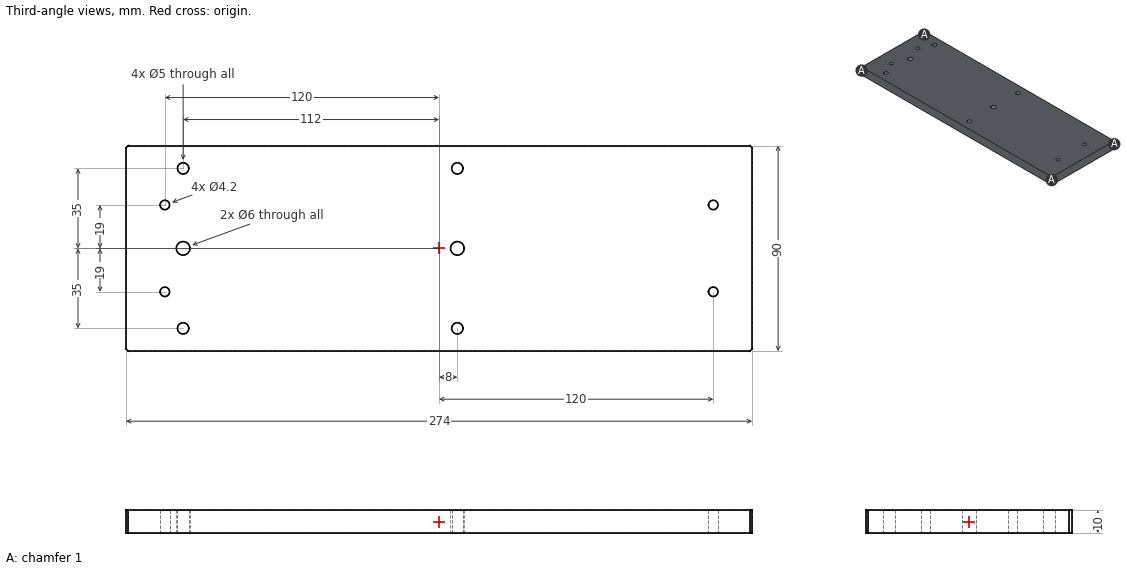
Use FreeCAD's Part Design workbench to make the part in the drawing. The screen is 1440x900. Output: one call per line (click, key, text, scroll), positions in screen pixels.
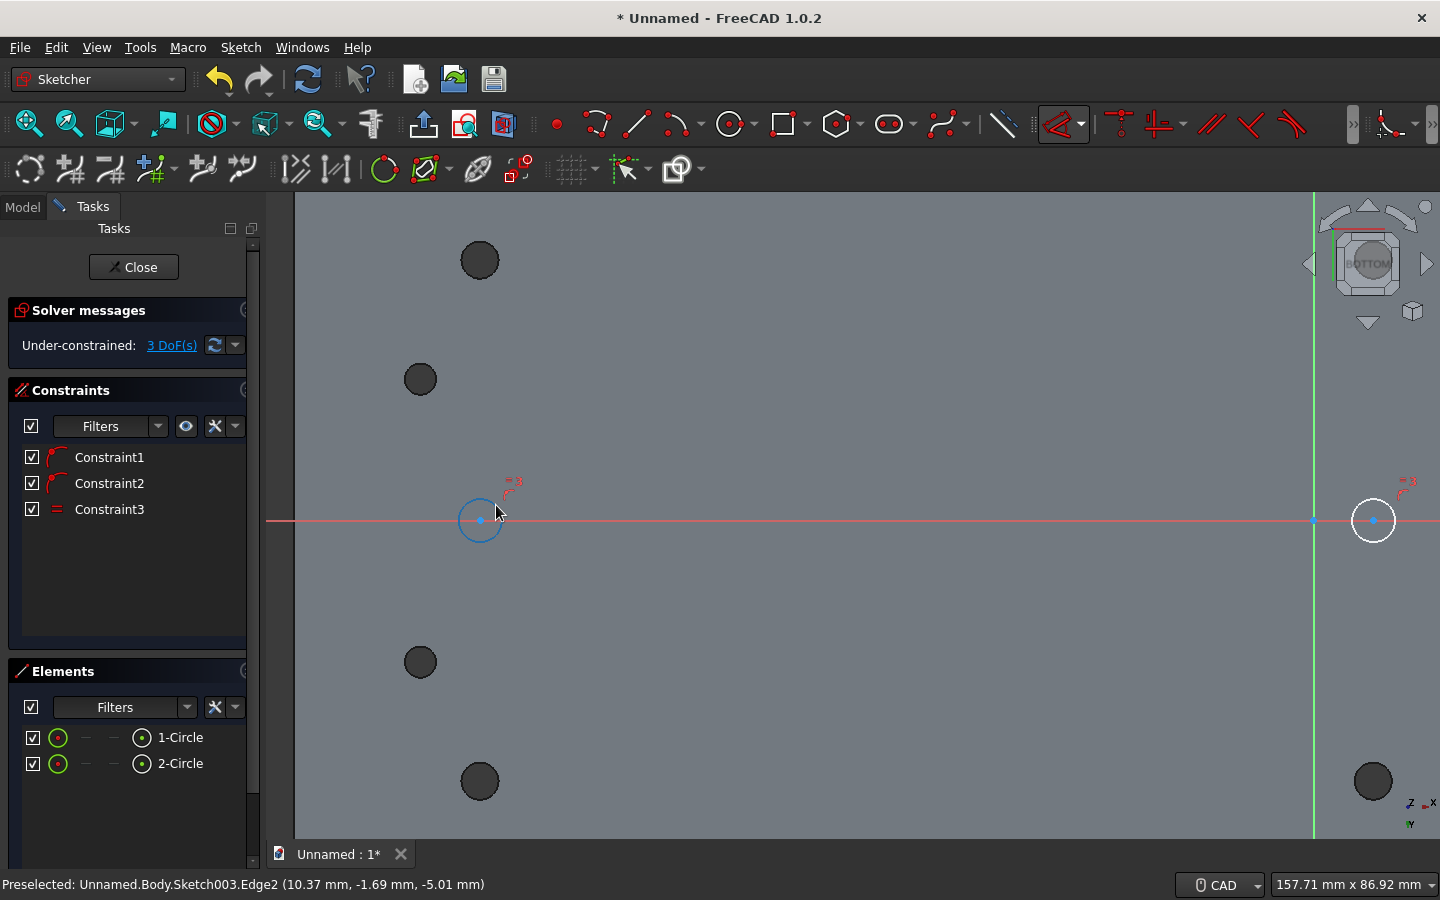
click(495, 505)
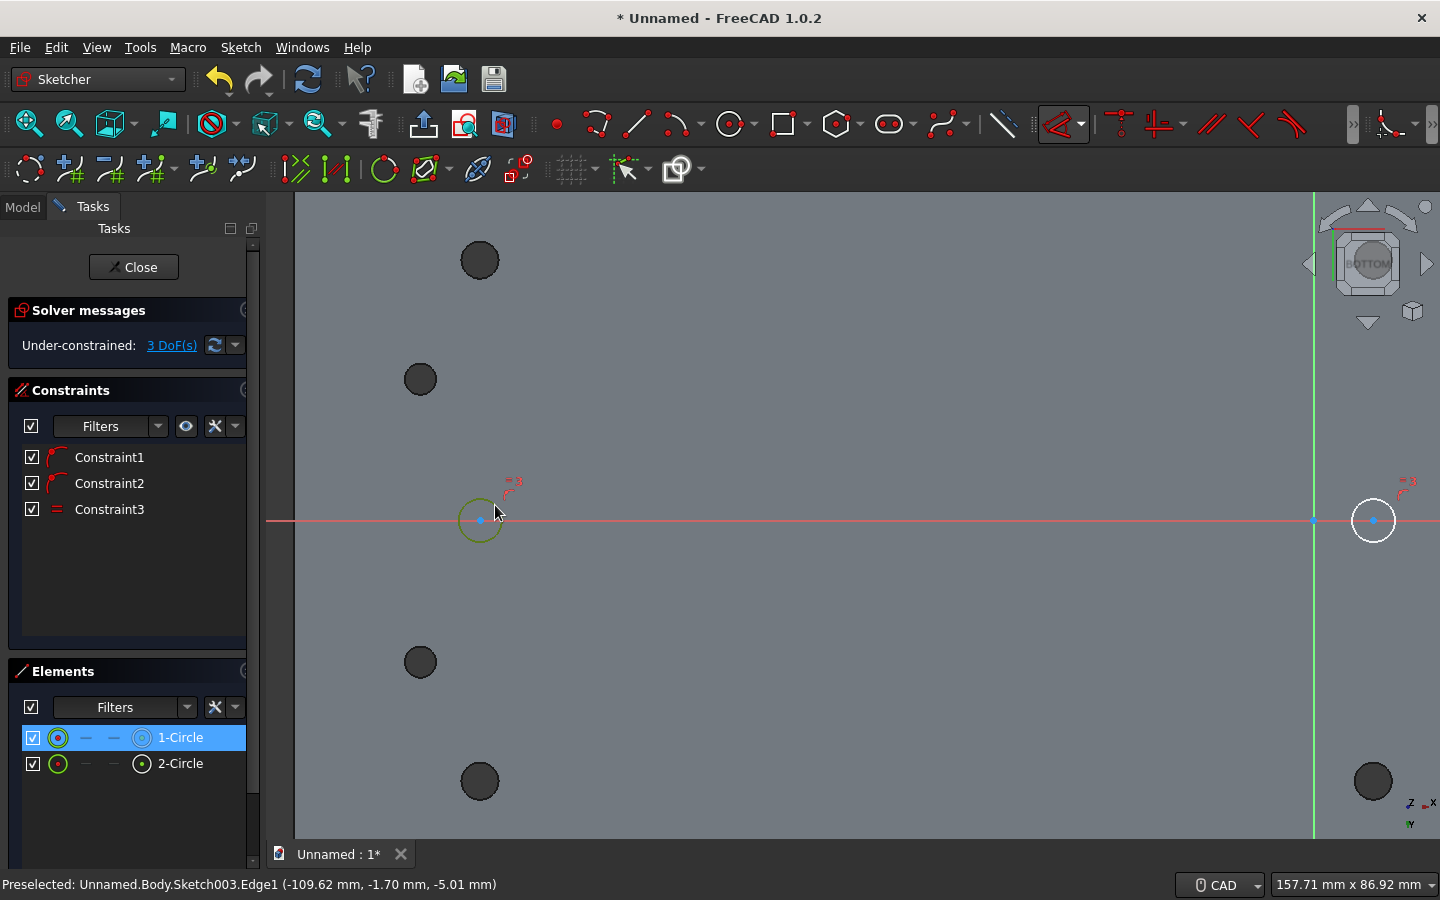
key(k)
key(o)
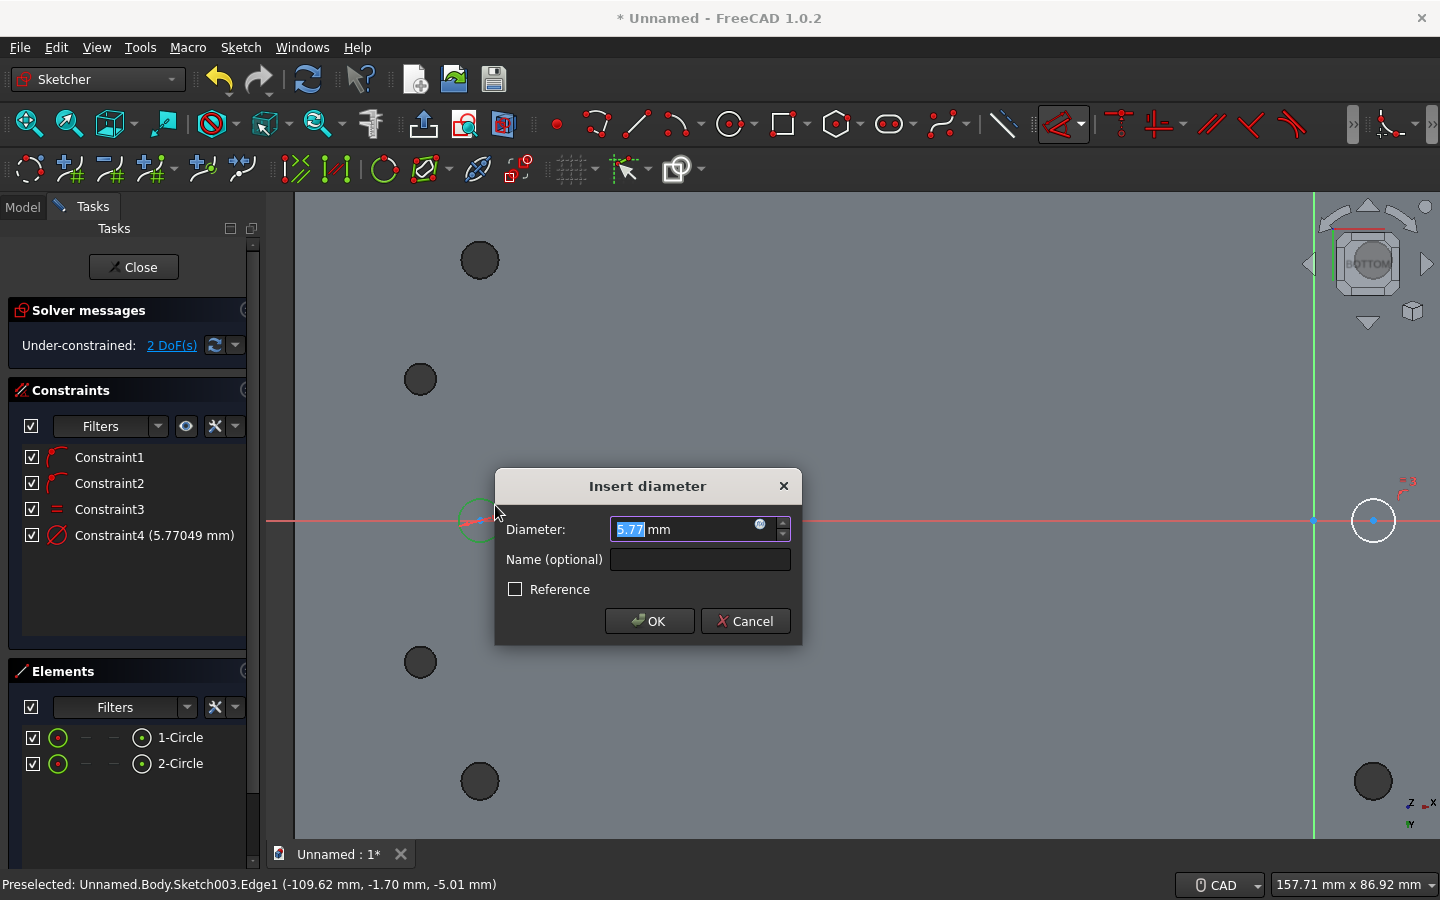
text(6)
key(Return)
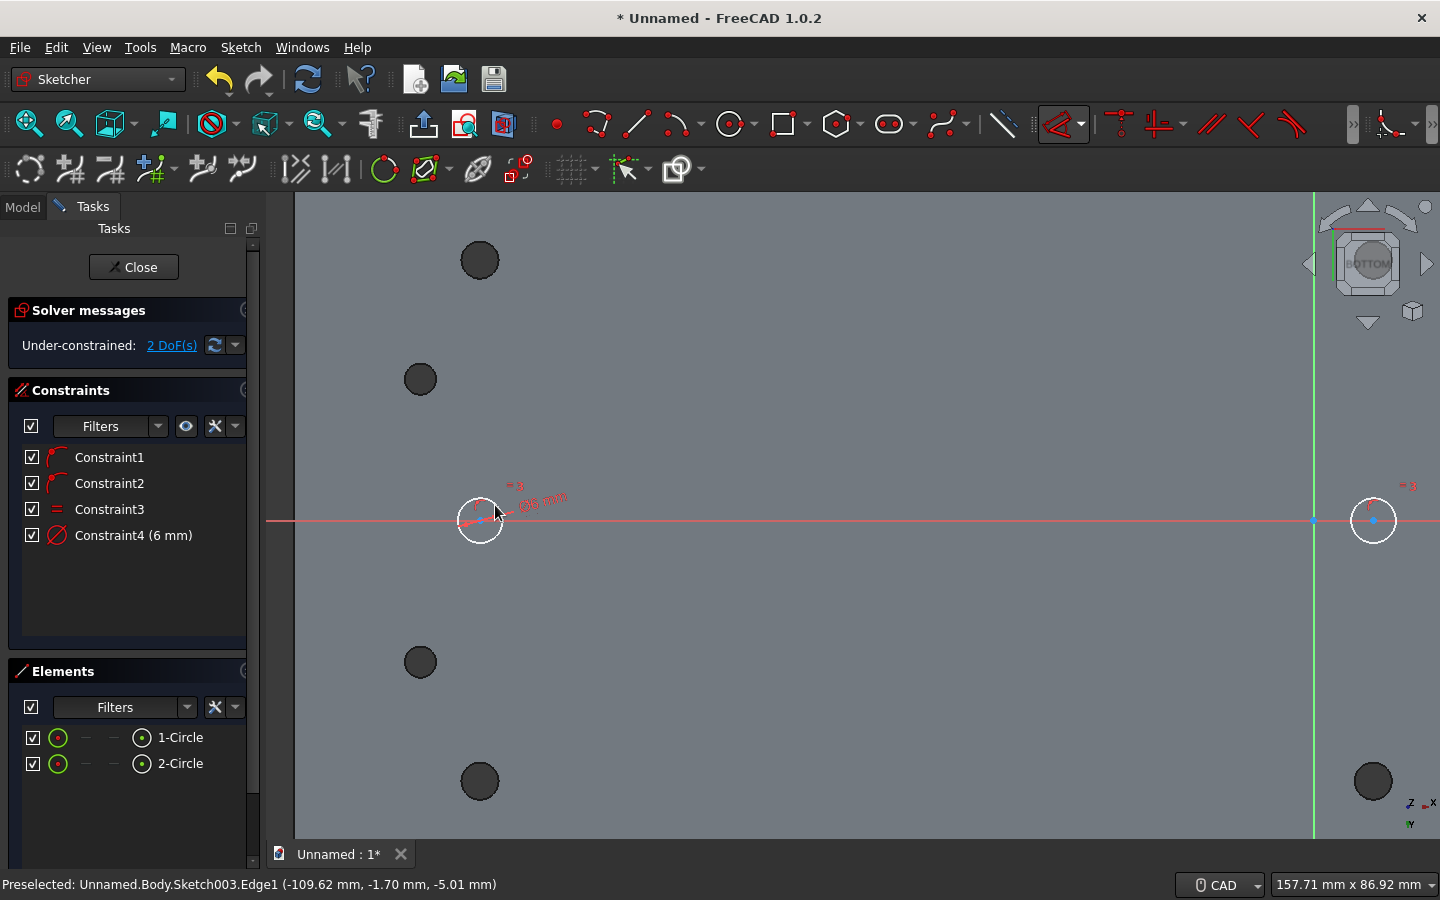
scroll(496, 505, down, 2)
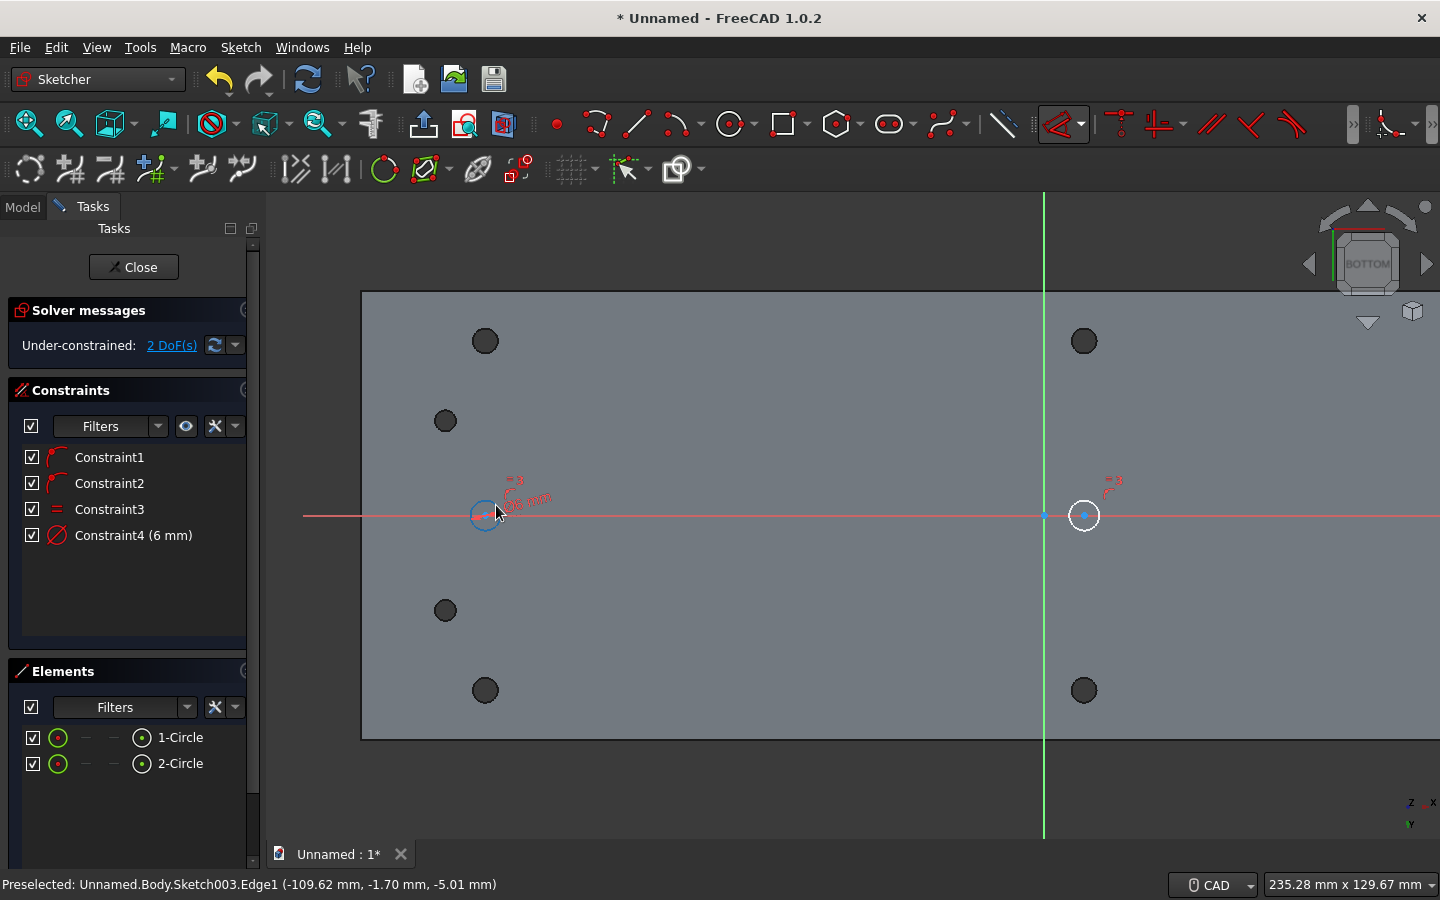
click(1084, 516)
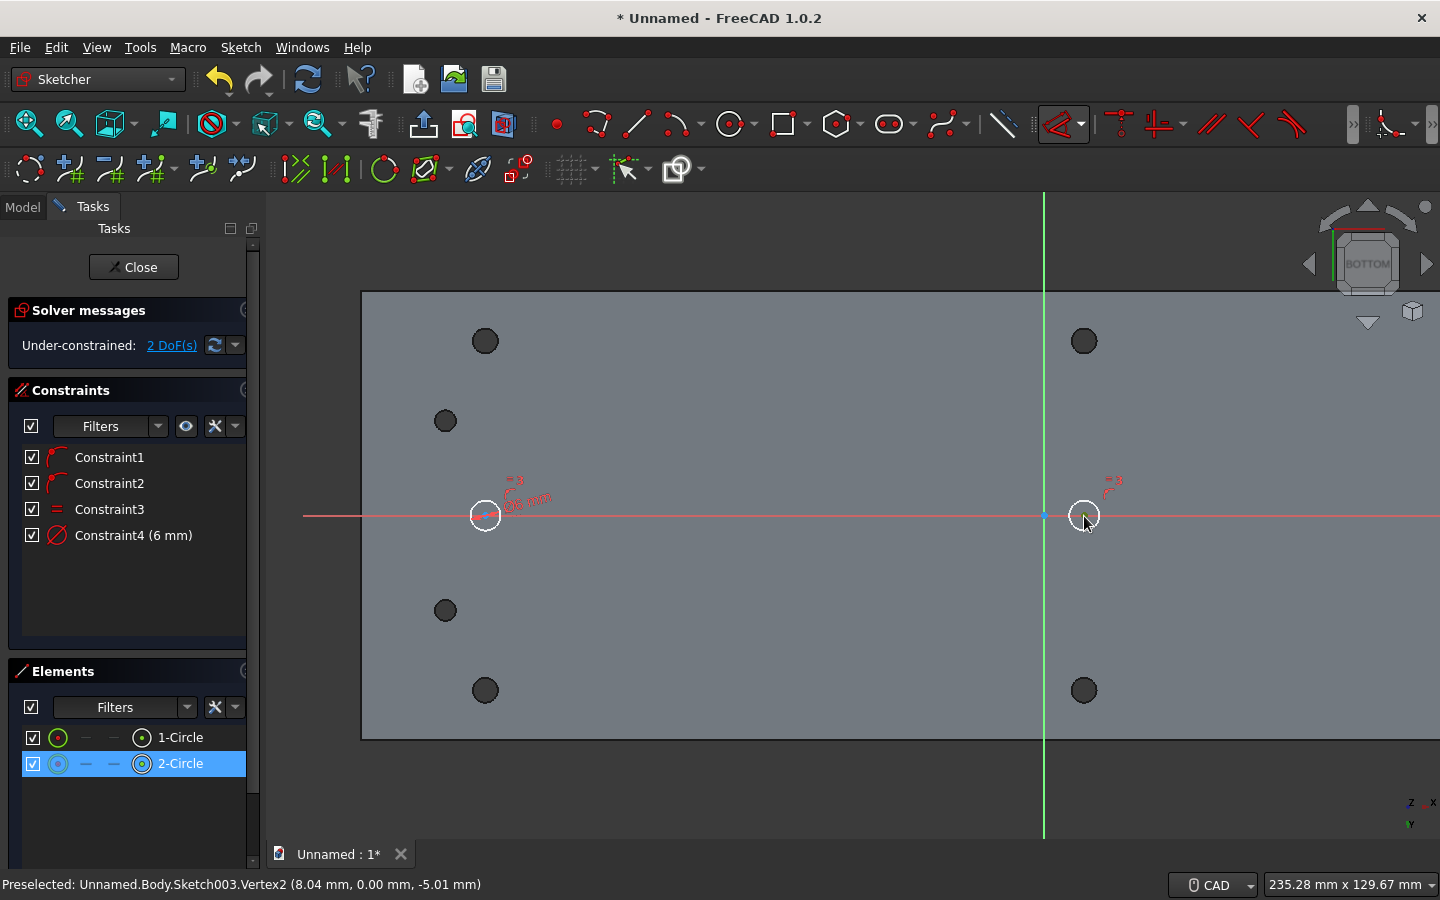
key(l)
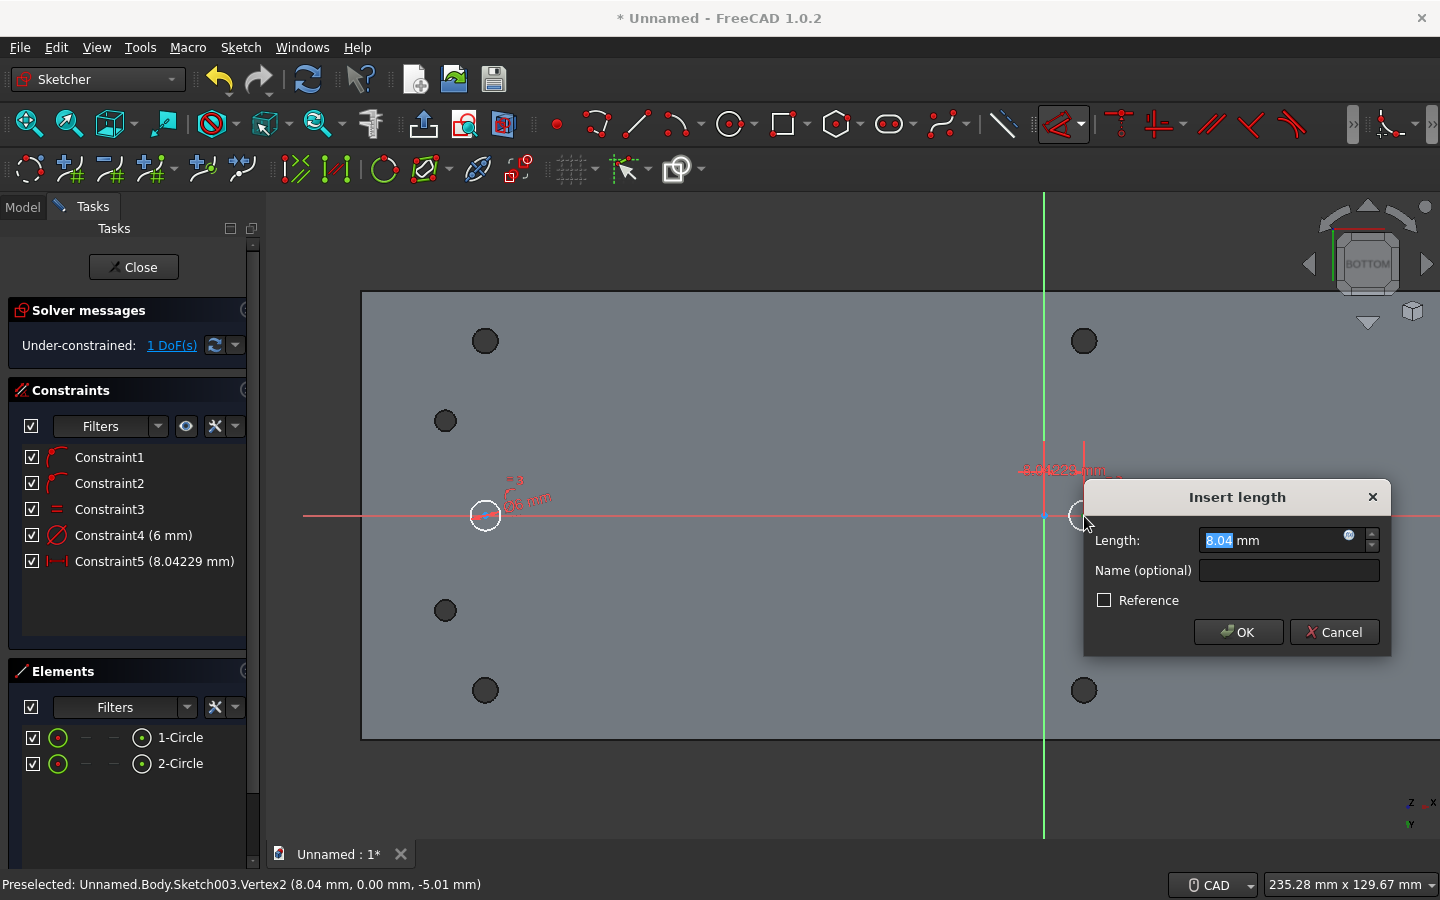
text(8)
key(Return)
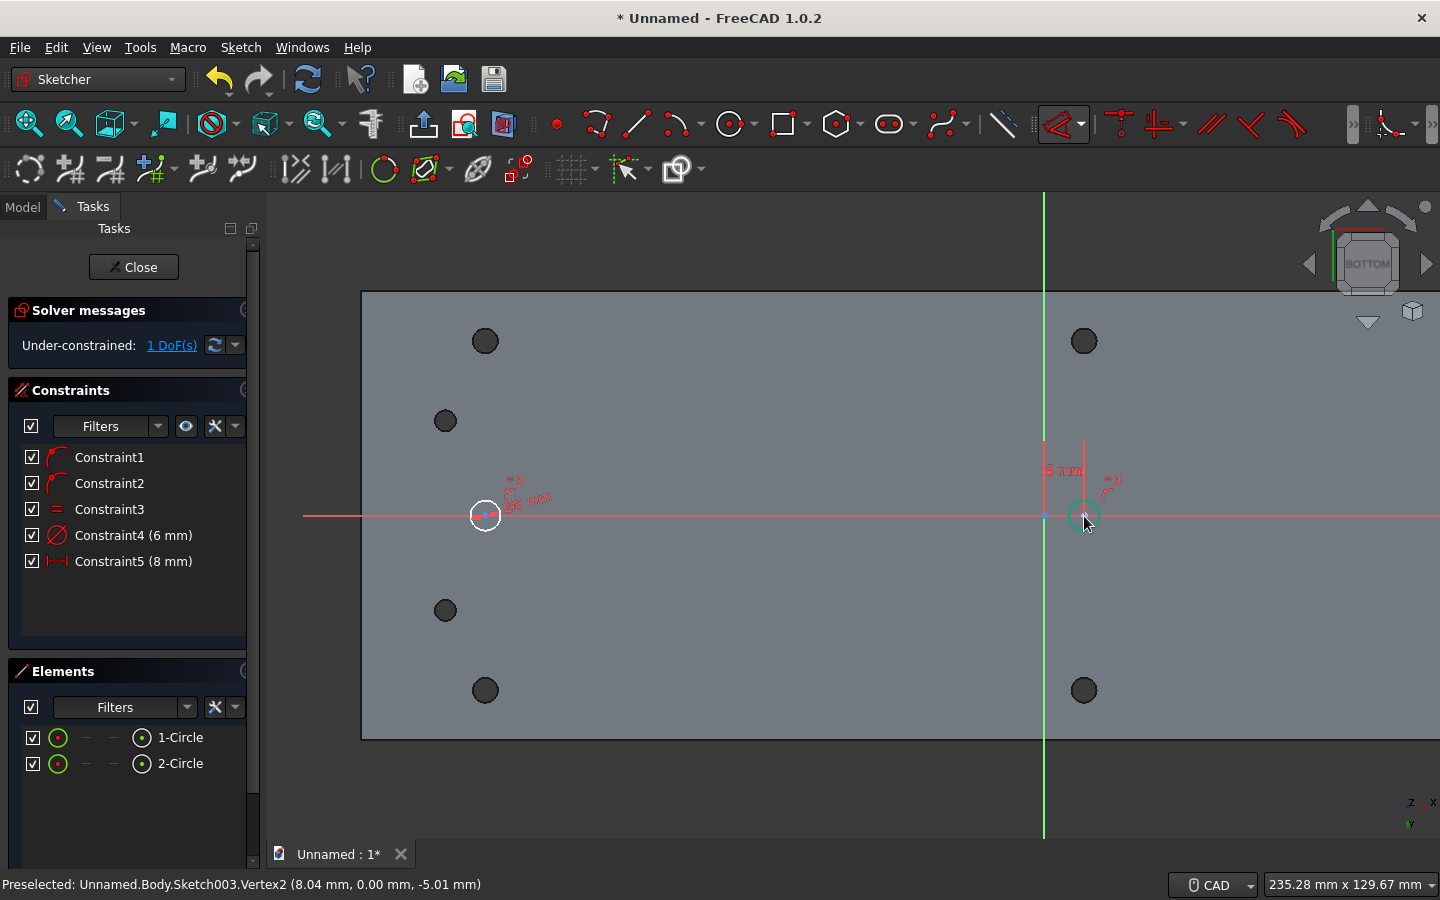
click(486, 516)